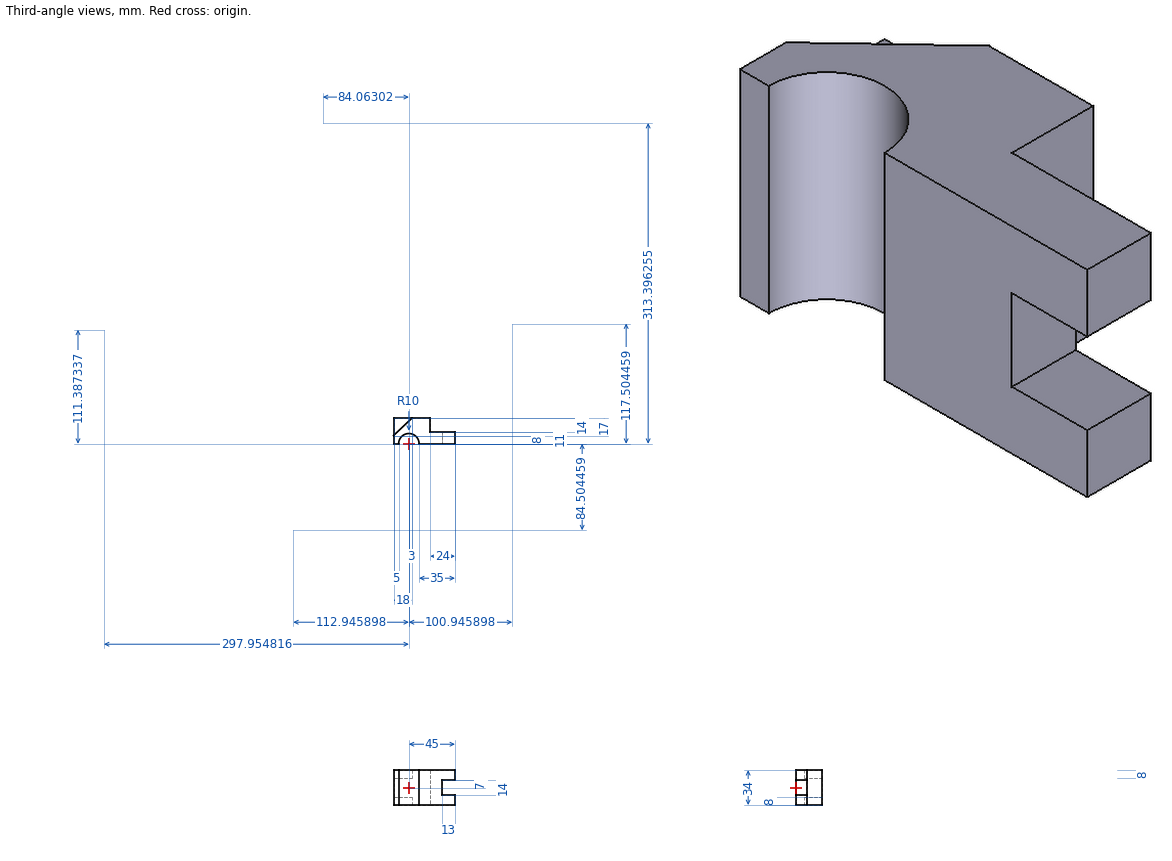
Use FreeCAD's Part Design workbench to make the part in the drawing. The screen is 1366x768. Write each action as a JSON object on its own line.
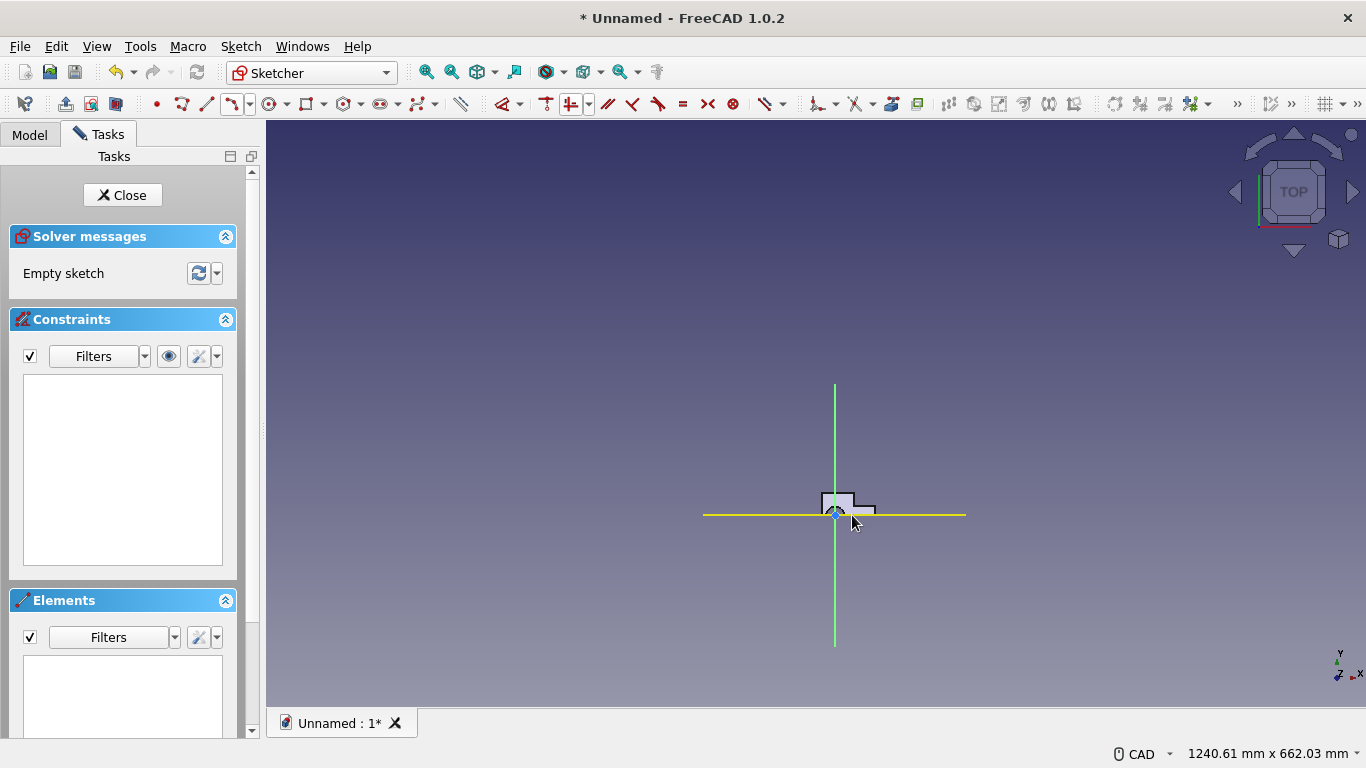
{"action": "left_click", "coordinate": [182, 104]}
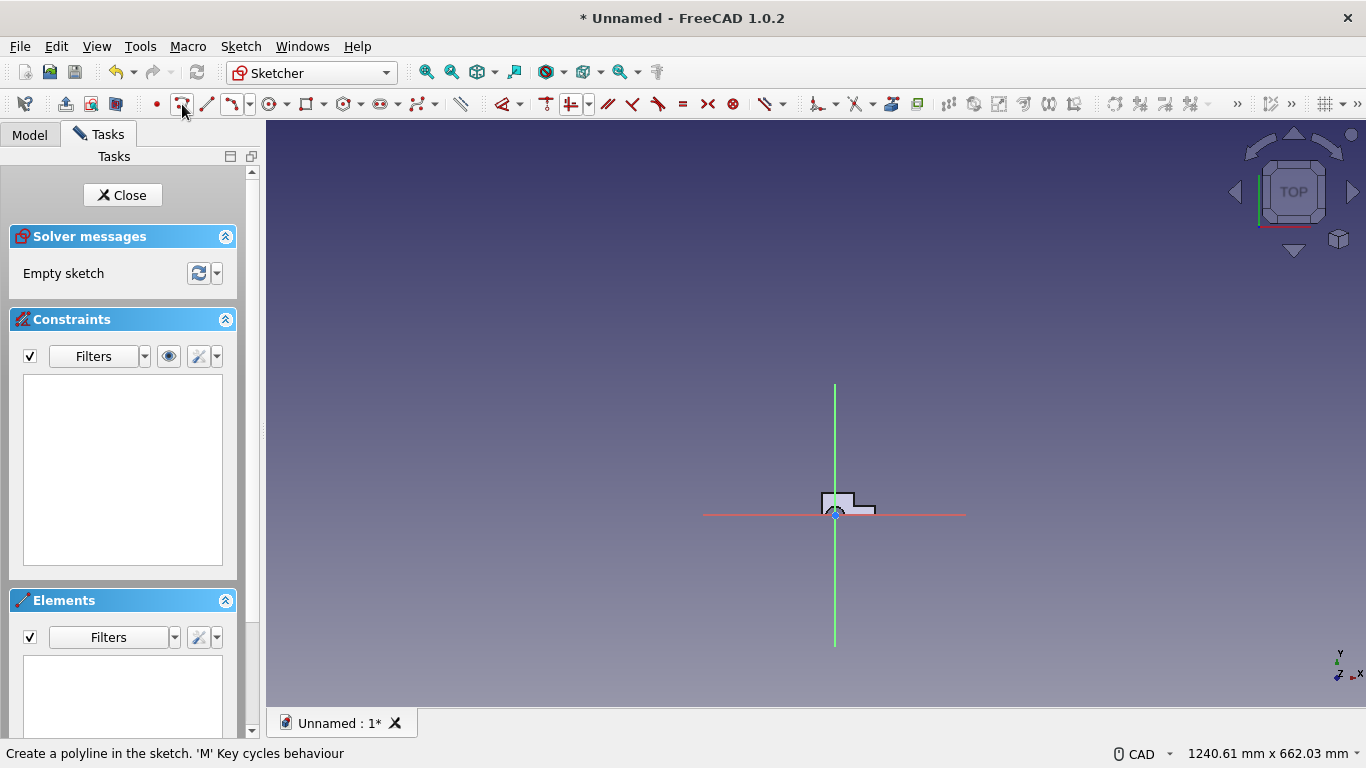
{"action": "left_click", "coordinate": [735, 590]}
{"action": "left_click", "coordinate": [925, 411]}
{"action": "left_click", "coordinate": [761, 238]}
{"action": "left_click", "coordinate": [571, 417]}
{"action": "left_click", "coordinate": [735, 591]}
{"action": "key", "text": "Escape"}
{"action": "key", "text": "Escape"}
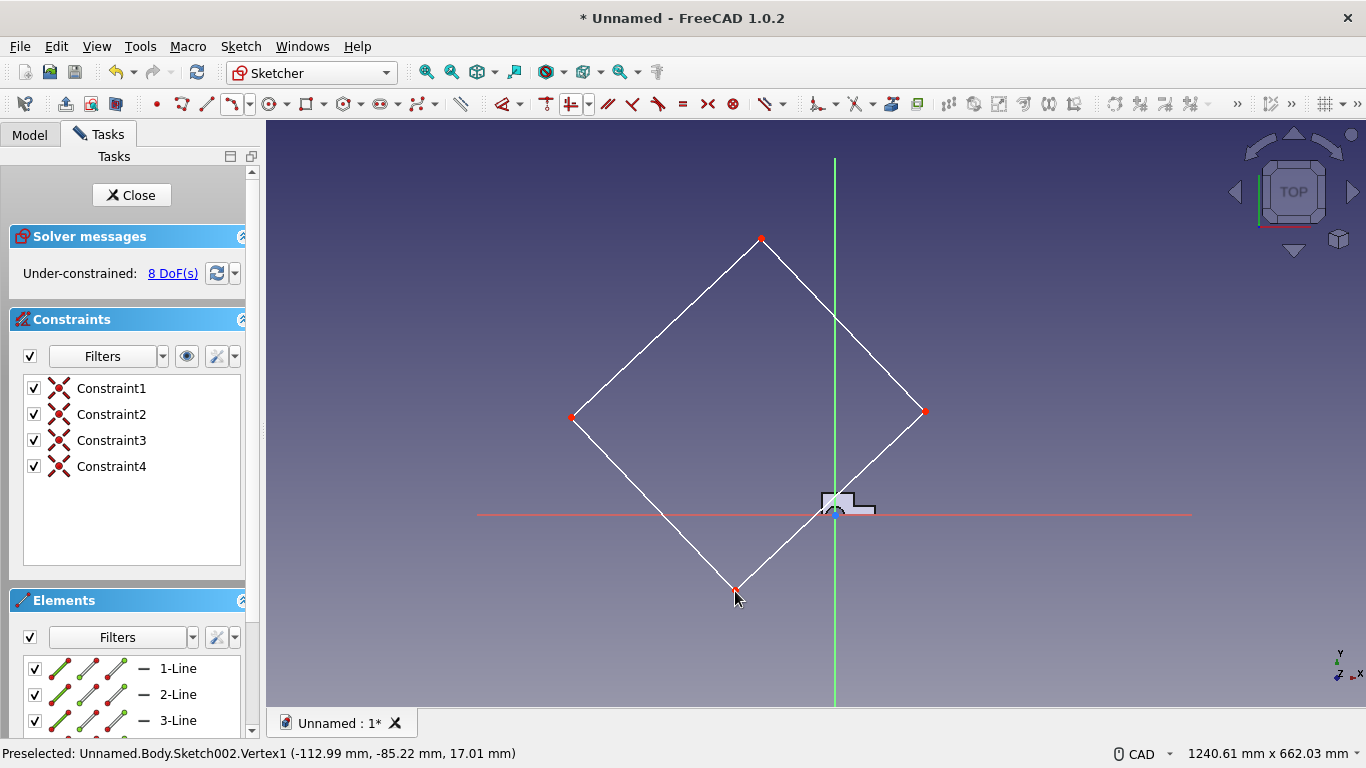
{"action": "left_click", "coordinate": [502, 104]}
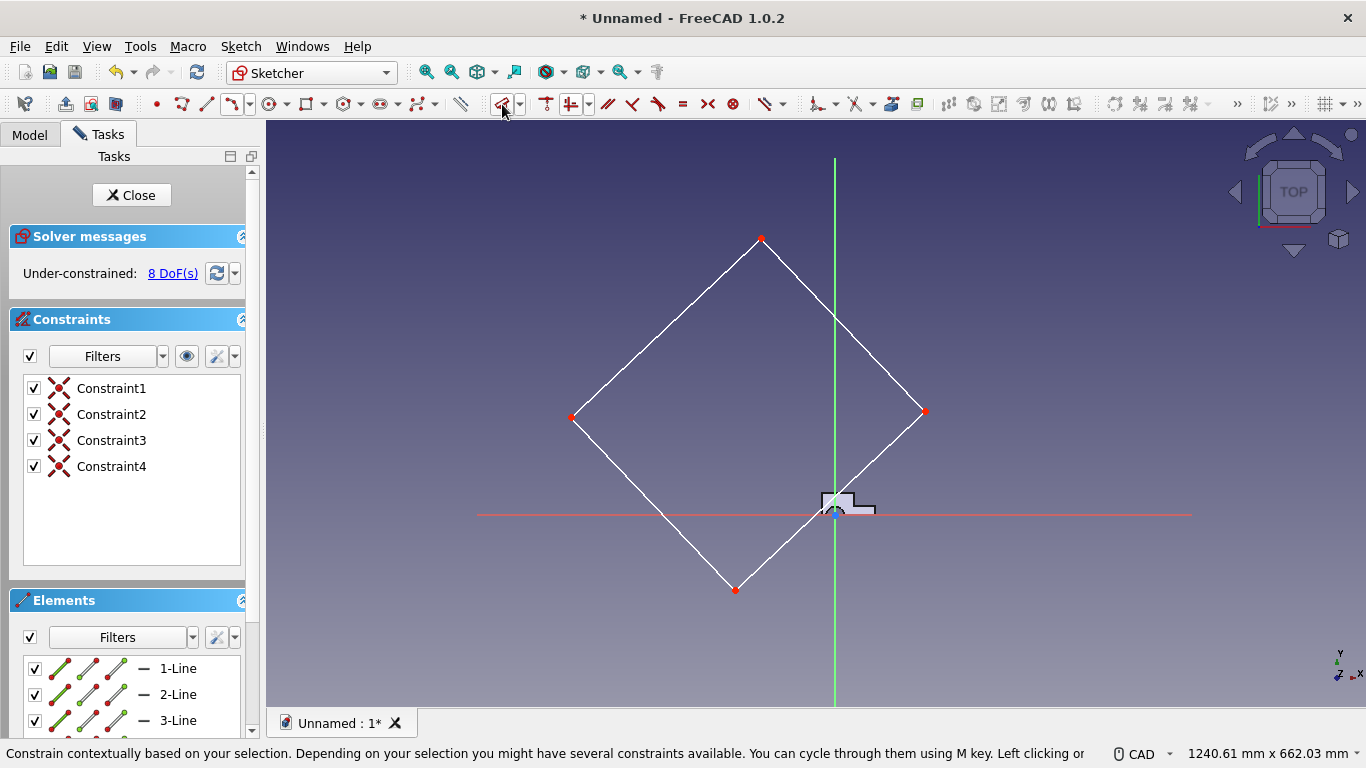
{"action": "left_click", "coordinate": [761, 239]}
{"action": "left_click", "coordinate": [798, 205]}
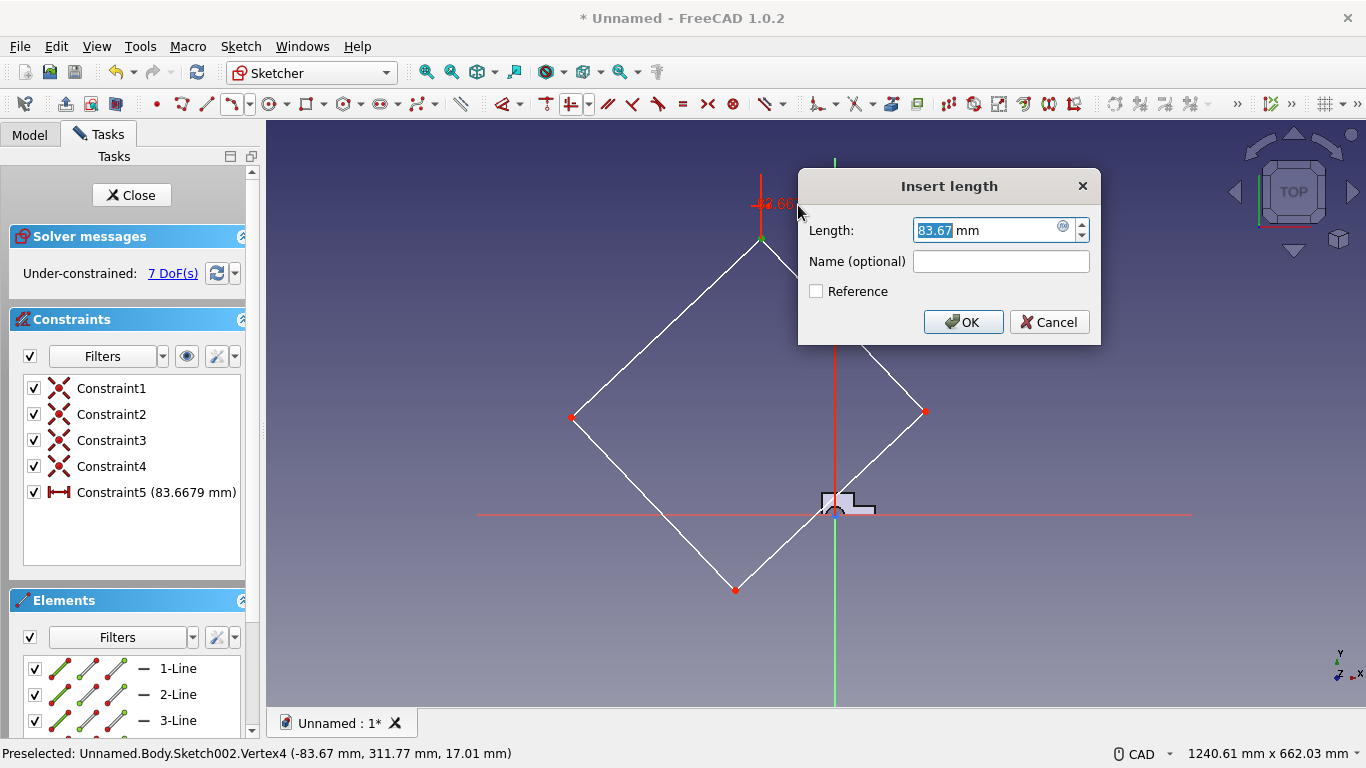
{"action": "type", "text": "84.06302"}
{"action": "key", "text": "Return"}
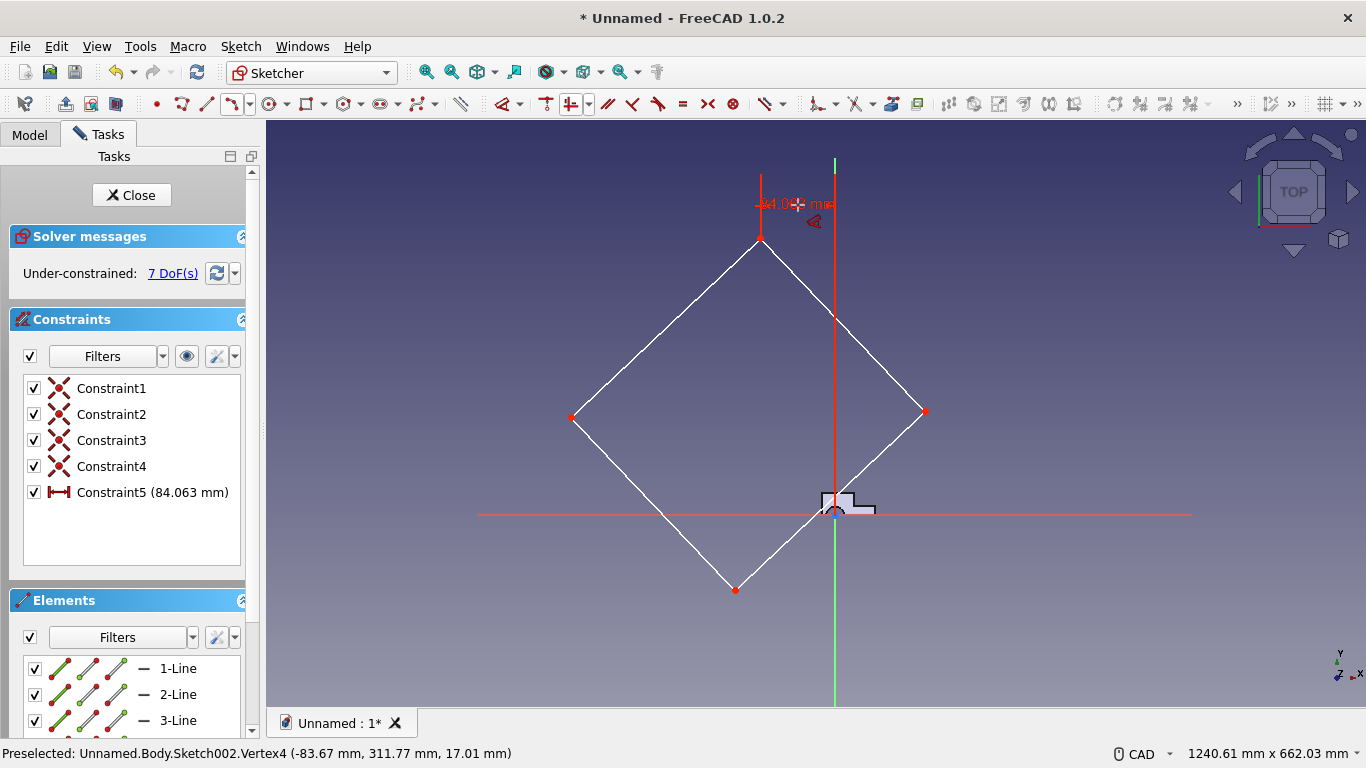
{"action": "left_click", "coordinate": [735, 591]}
{"action": "left_click", "coordinate": [869, 553]}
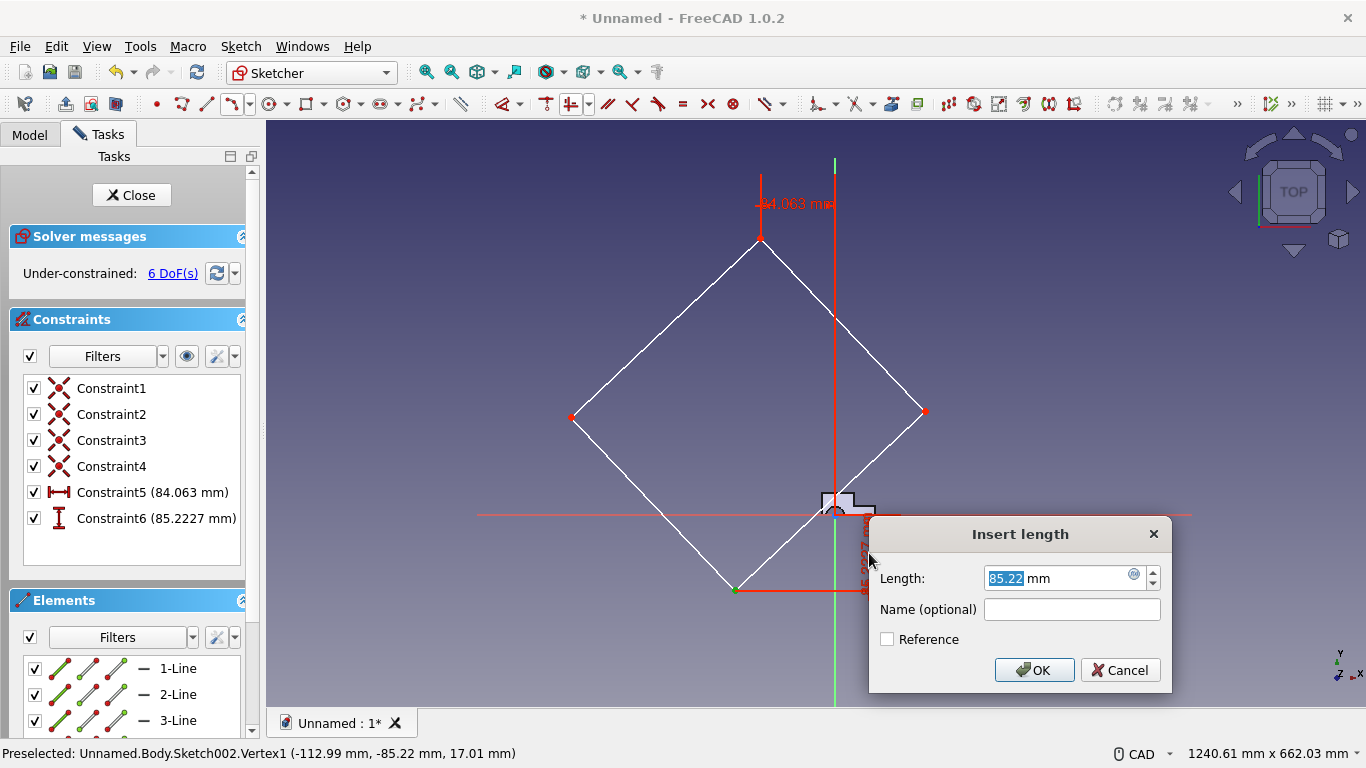
{"action": "type", "text": "84.504459"}
{"action": "key", "text": "Return"}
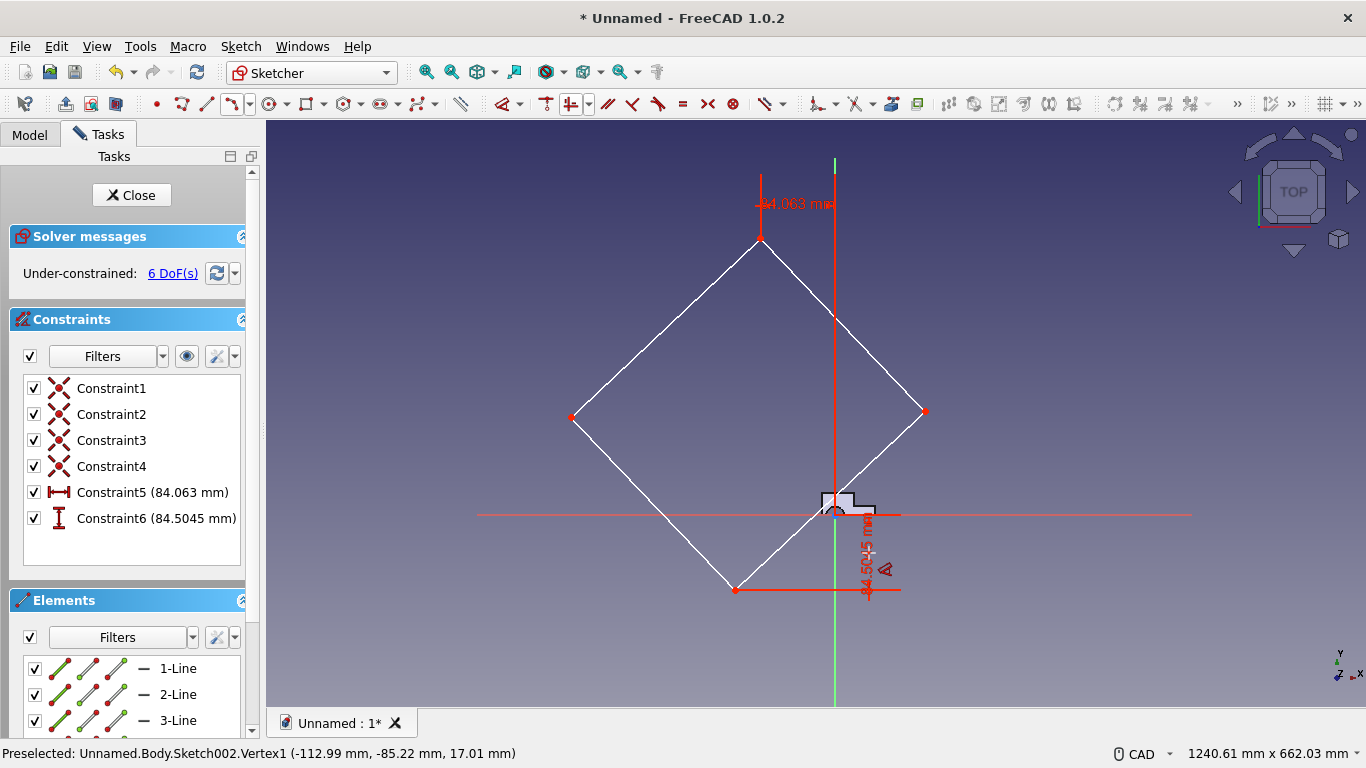
{"action": "left_click", "coordinate": [735, 590]}
{"action": "left_click", "coordinate": [785, 624]}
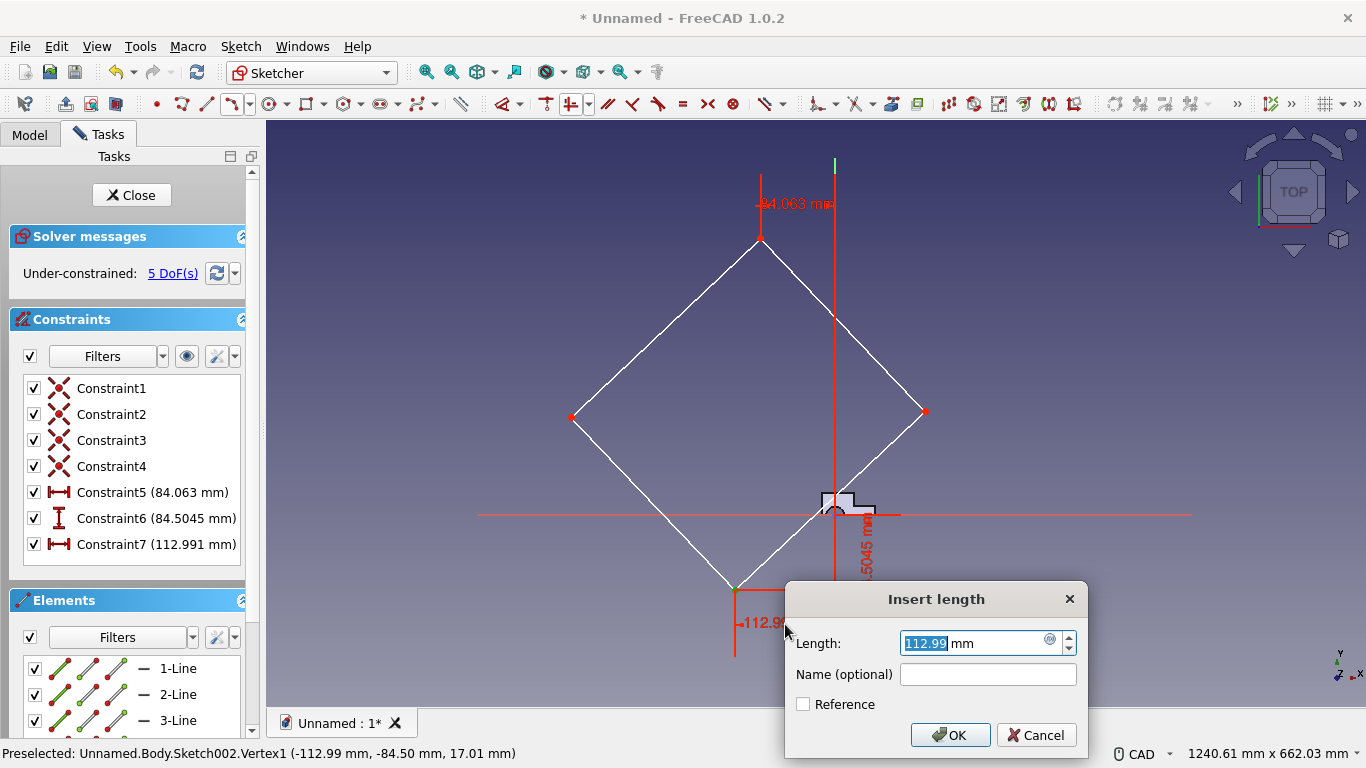
{"action": "type", "text": "112.945898"}
{"action": "key", "text": "Return"}